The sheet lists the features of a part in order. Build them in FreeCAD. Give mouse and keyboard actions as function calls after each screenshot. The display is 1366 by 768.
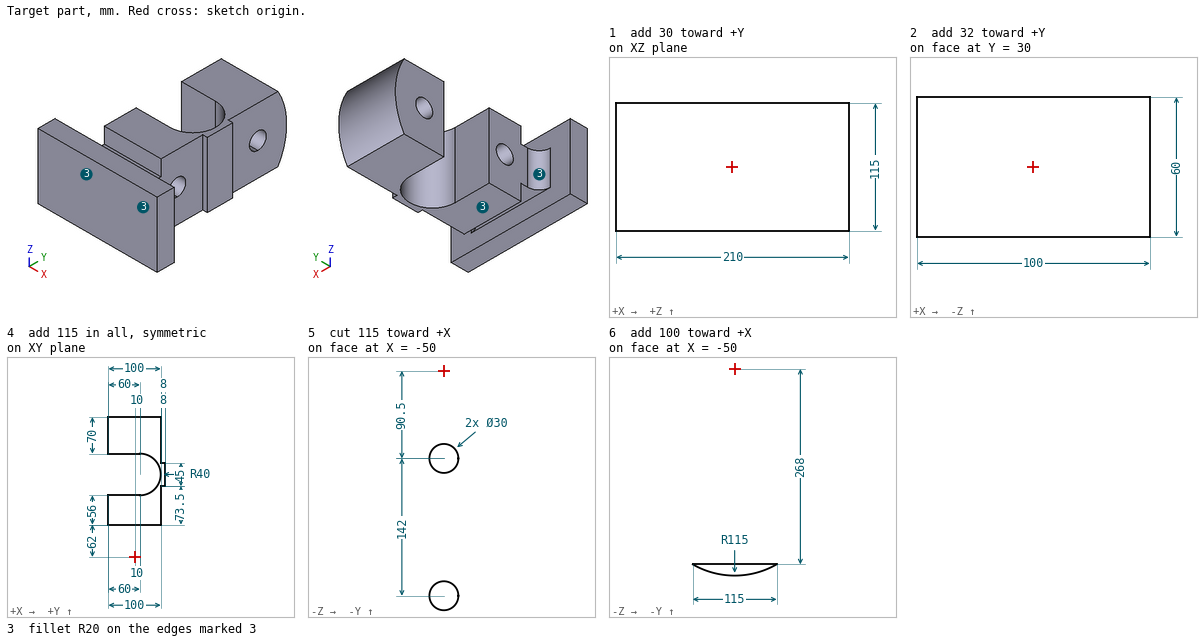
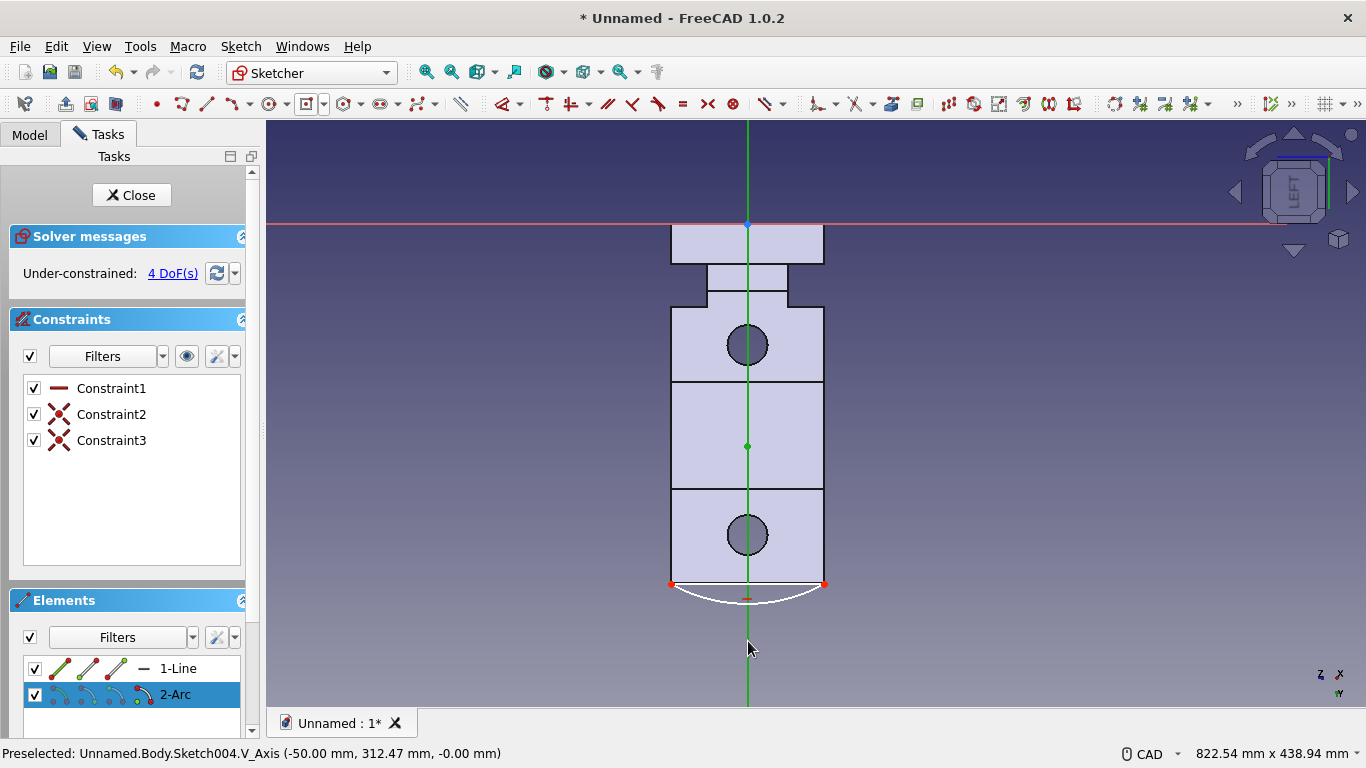
key(c)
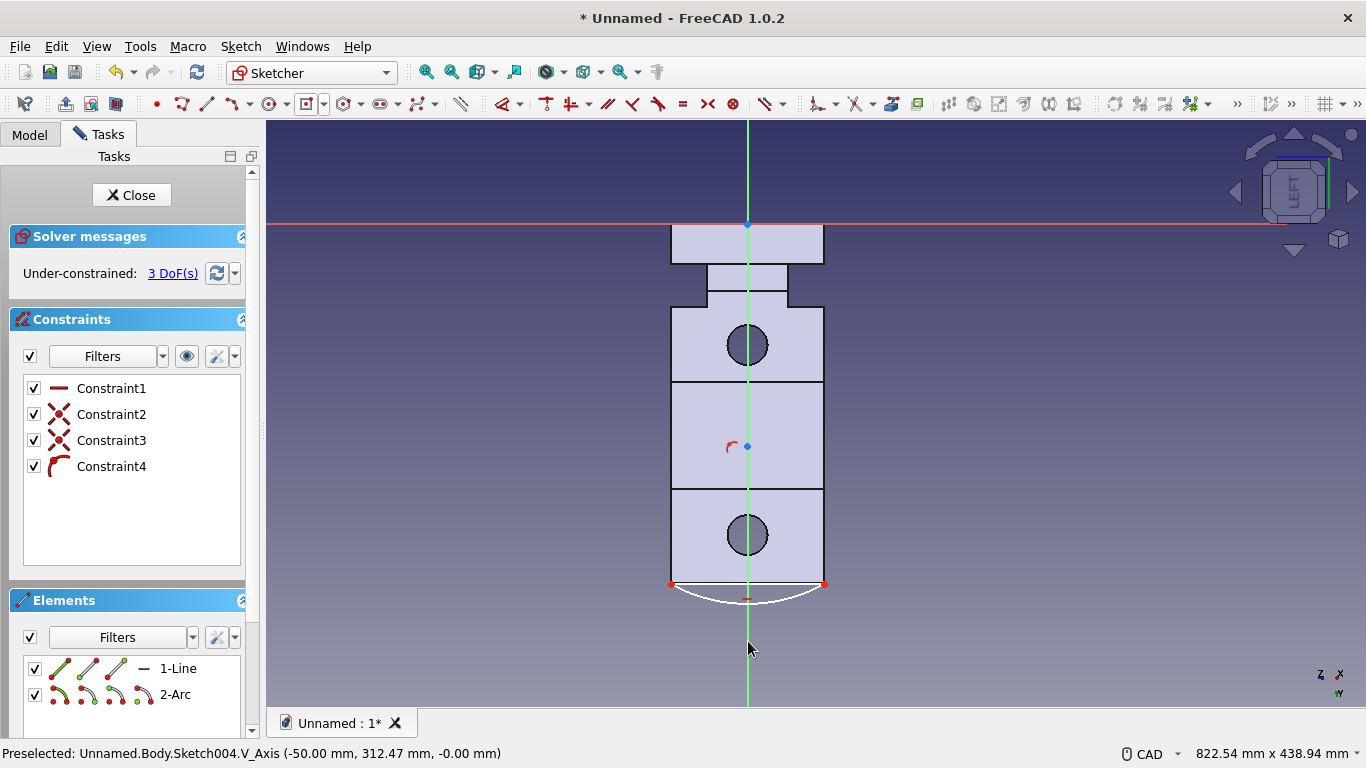
key(d)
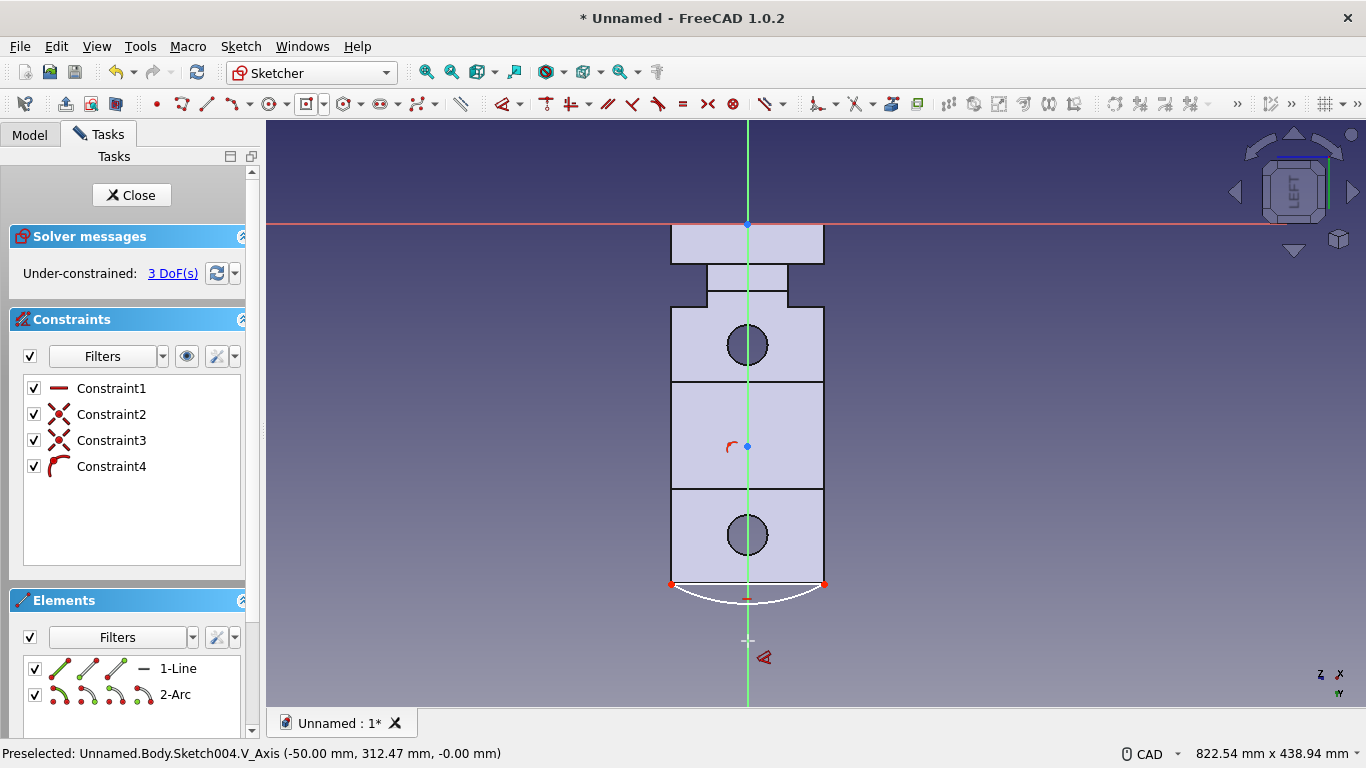
click(716, 601)
click(710, 632)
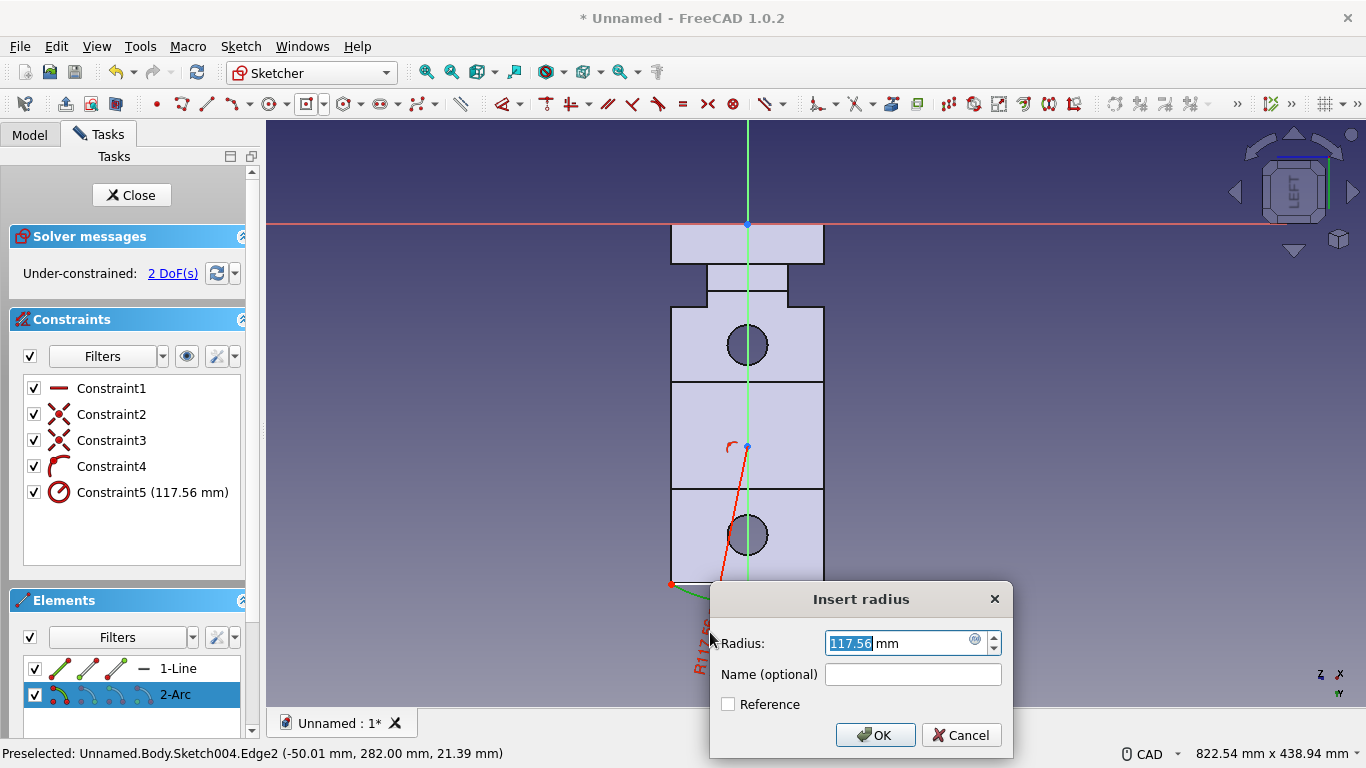
text(115)
key(Return)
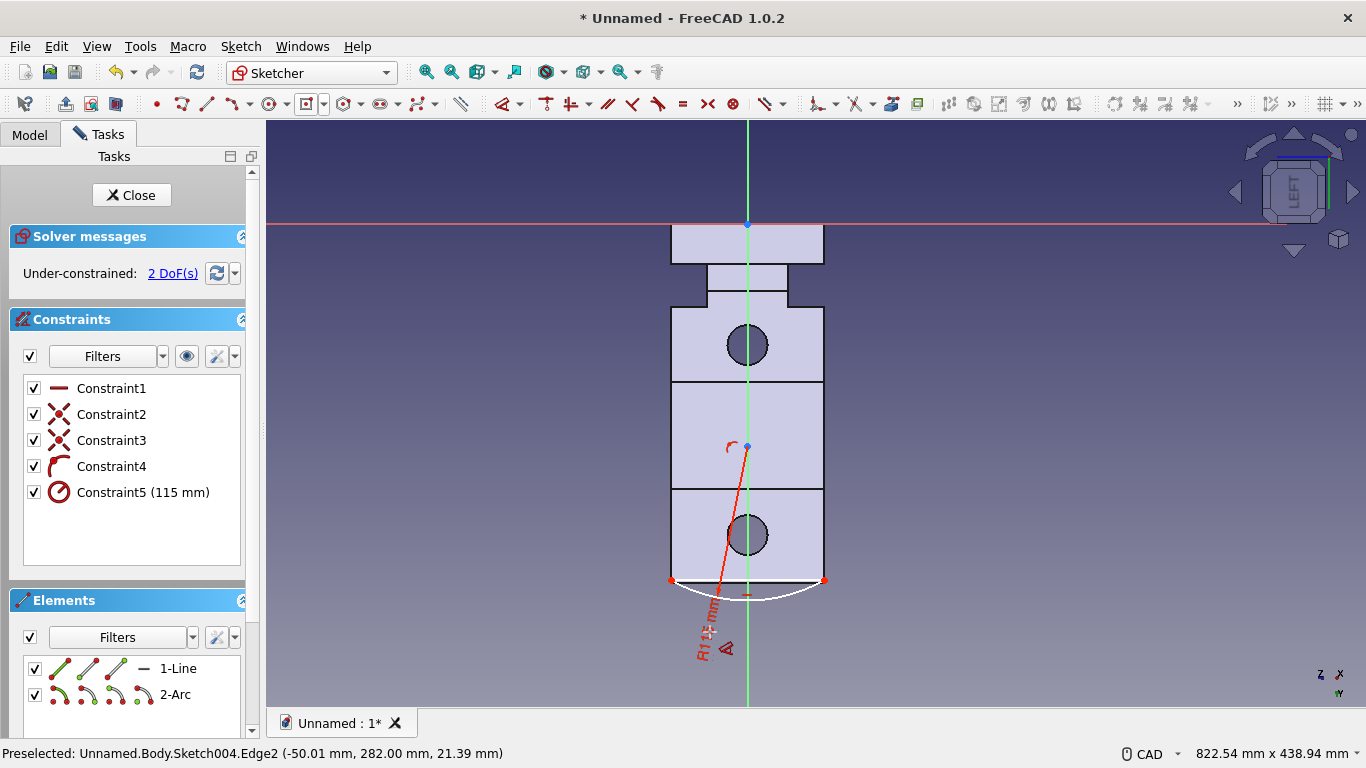
click(778, 580)
click(783, 614)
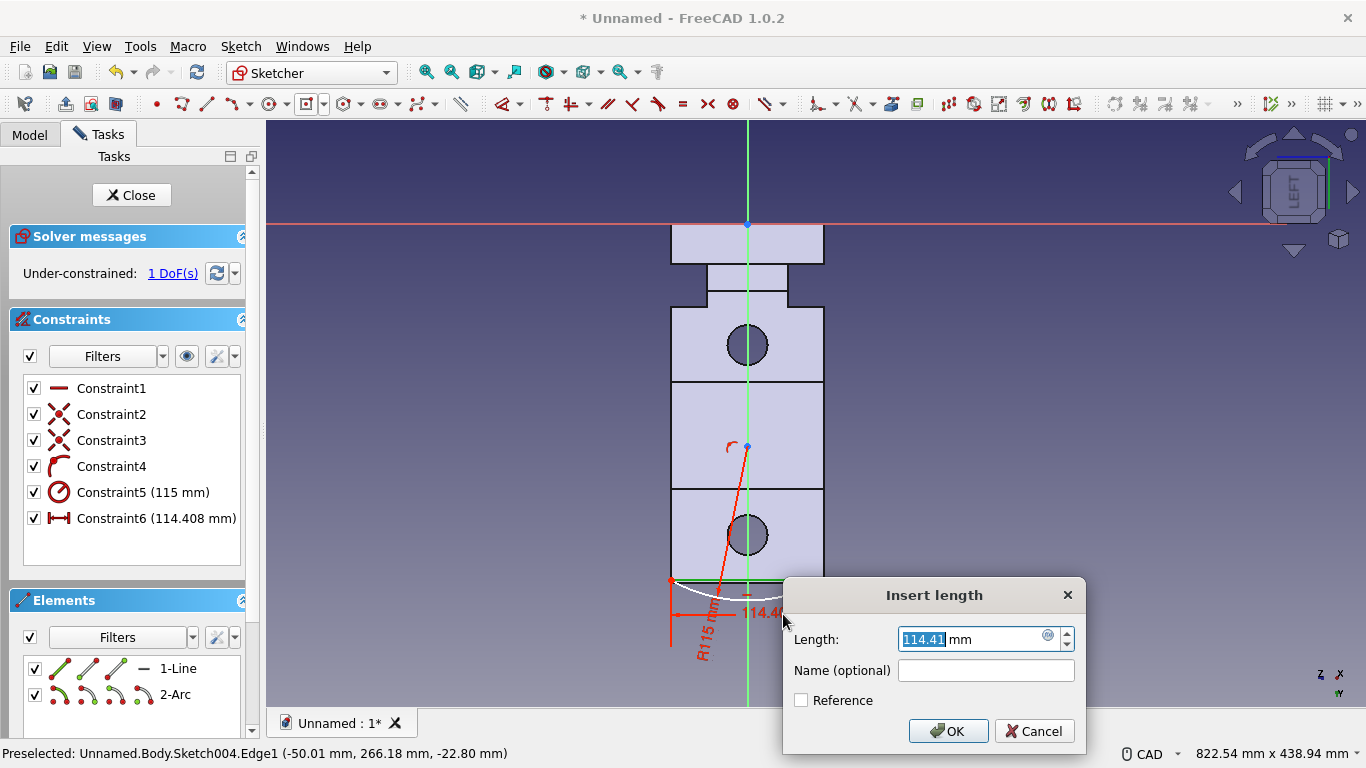
text(115)
key(Return)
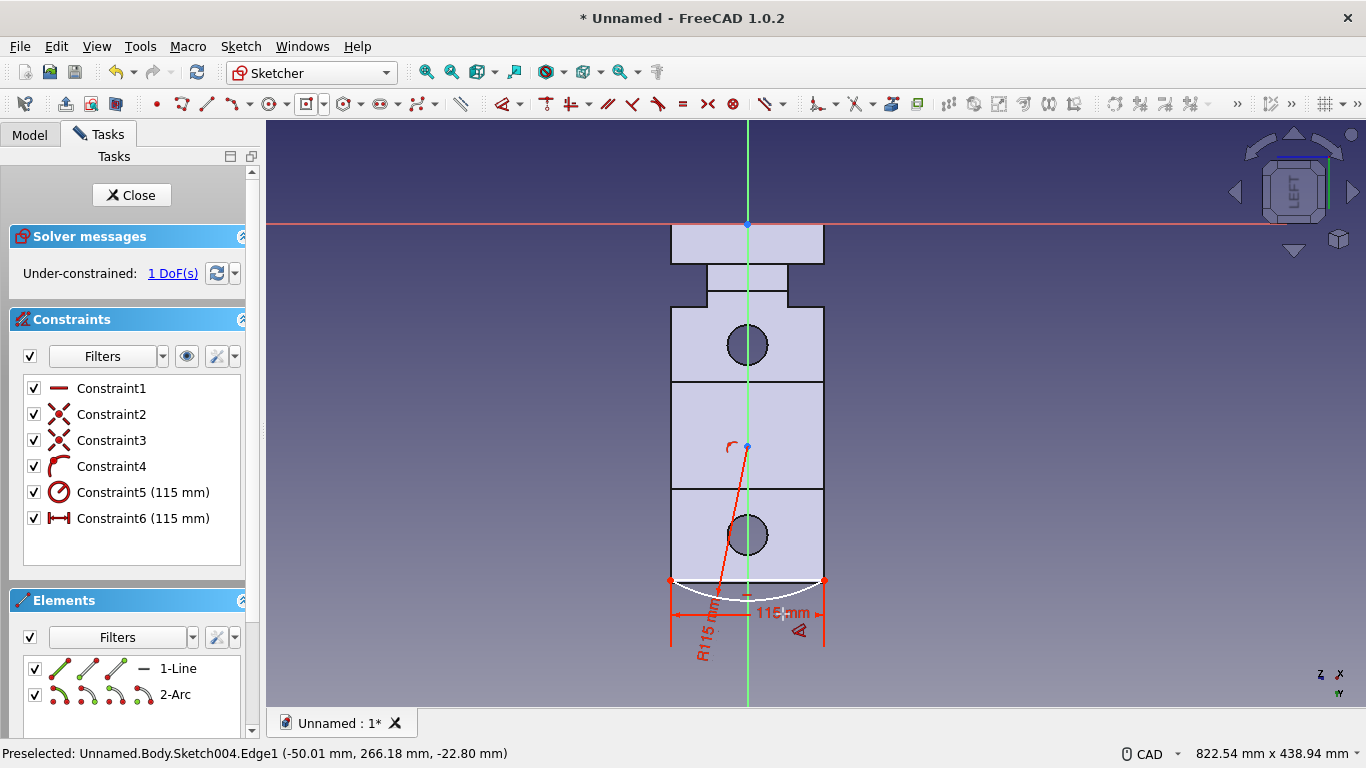
click(824, 580)
click(858, 402)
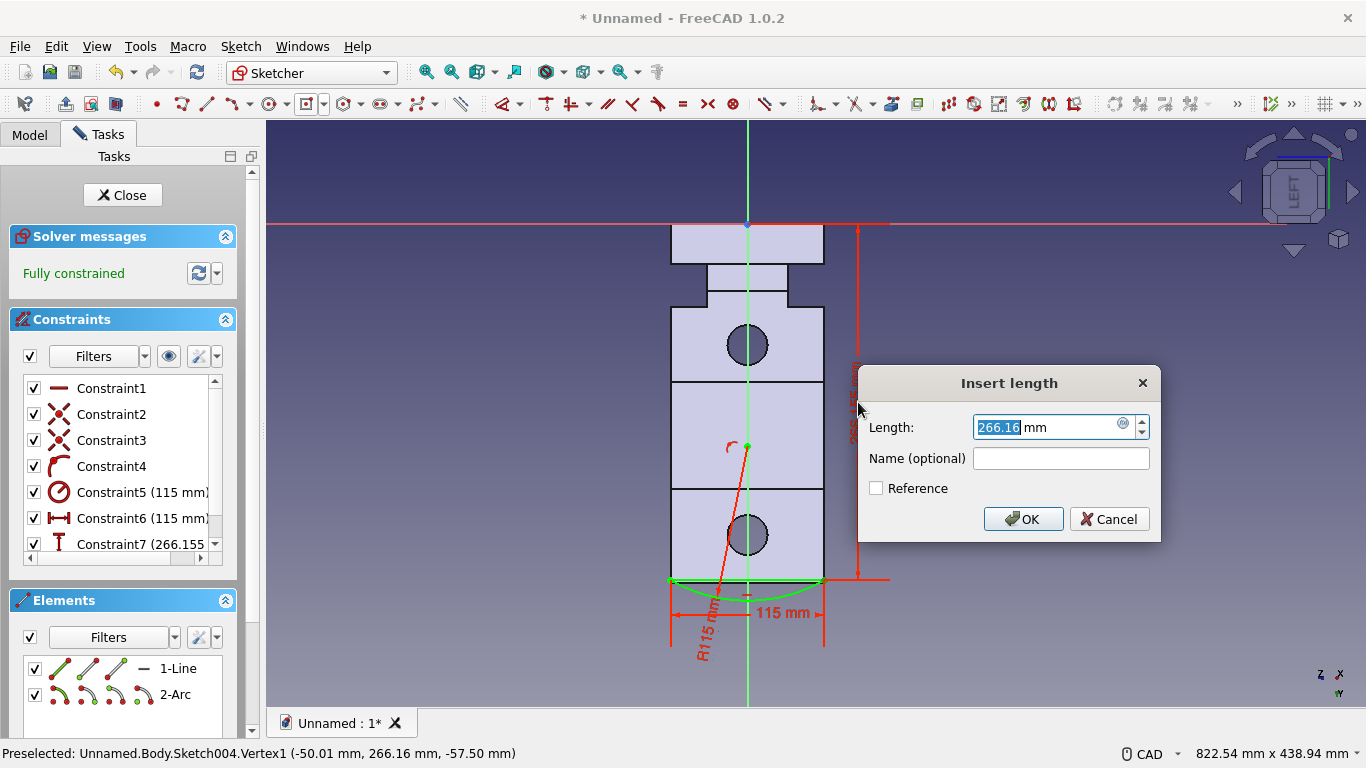
text(268)
key(Return)
key(Escape)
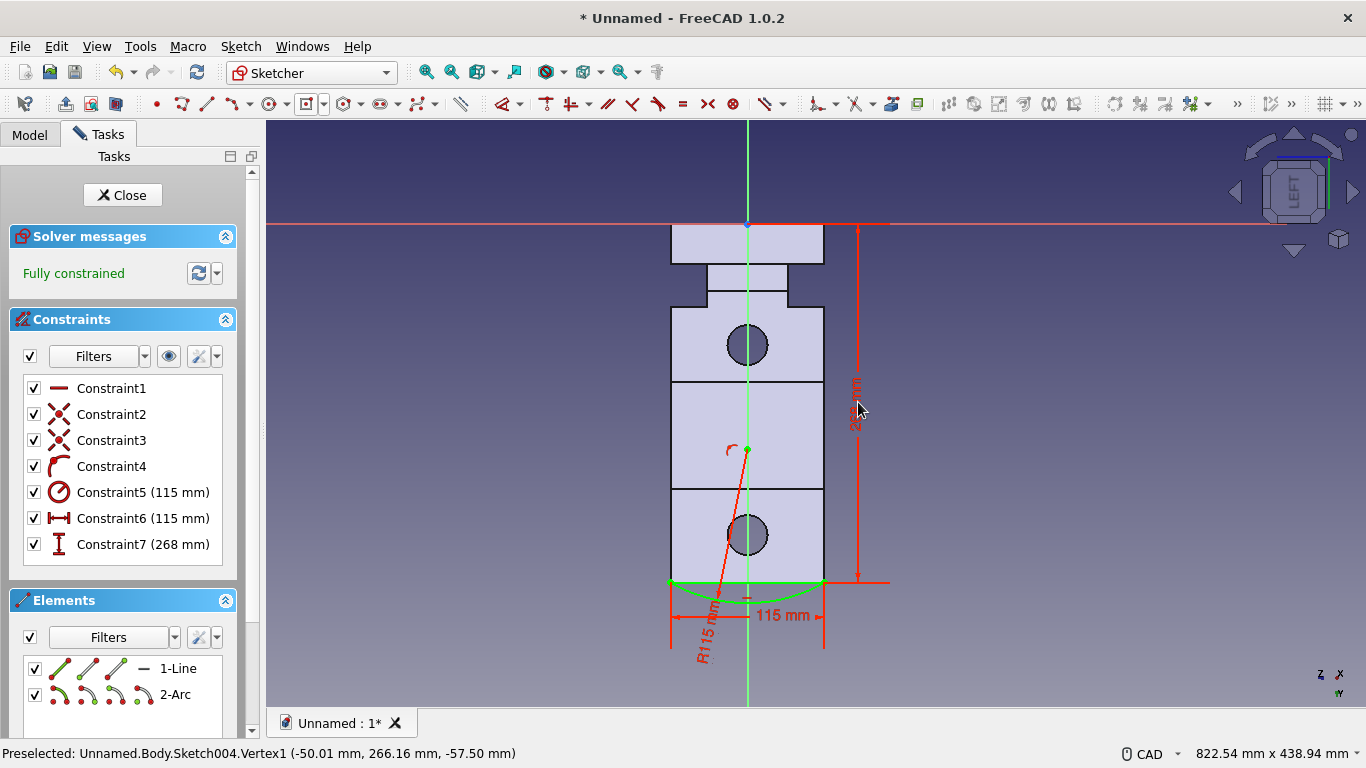
click(123, 195)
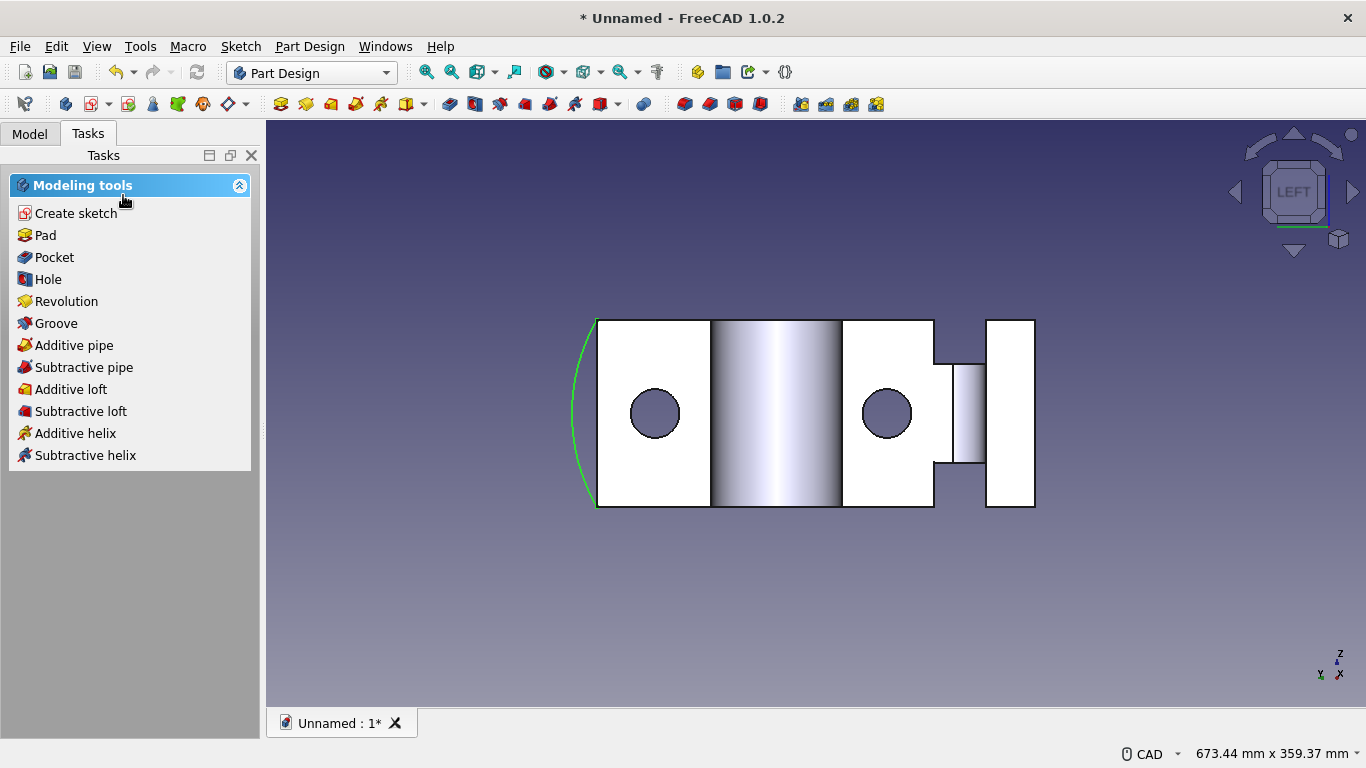
click(281, 104)